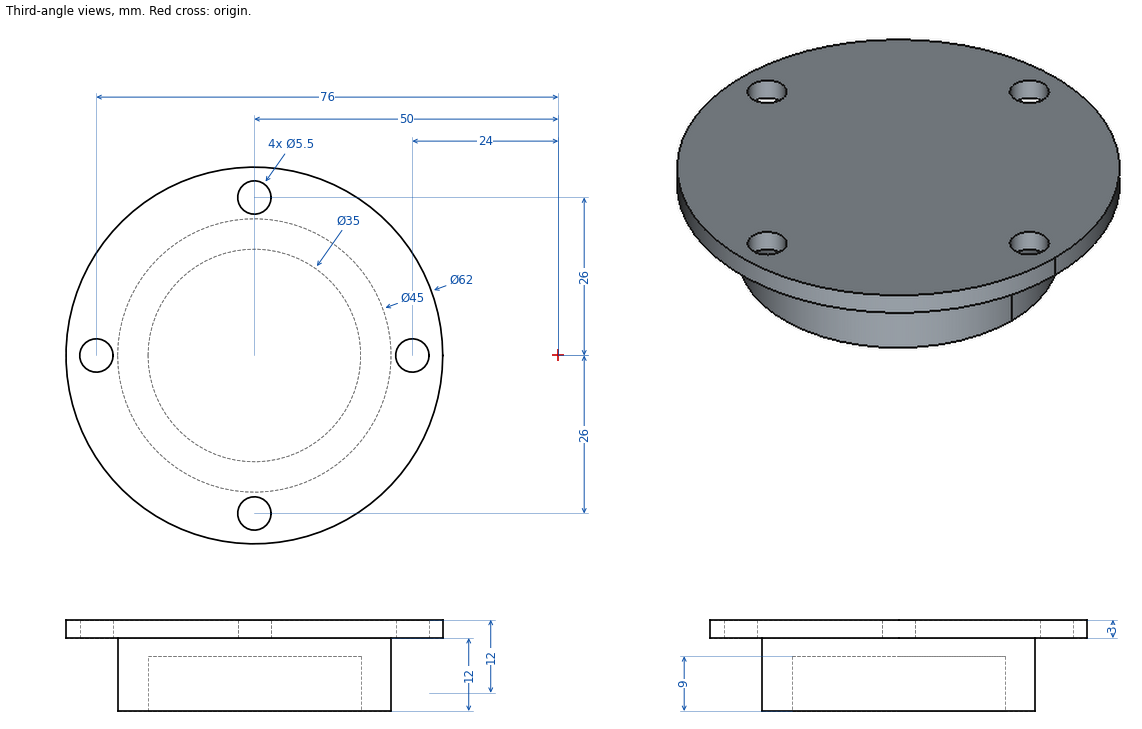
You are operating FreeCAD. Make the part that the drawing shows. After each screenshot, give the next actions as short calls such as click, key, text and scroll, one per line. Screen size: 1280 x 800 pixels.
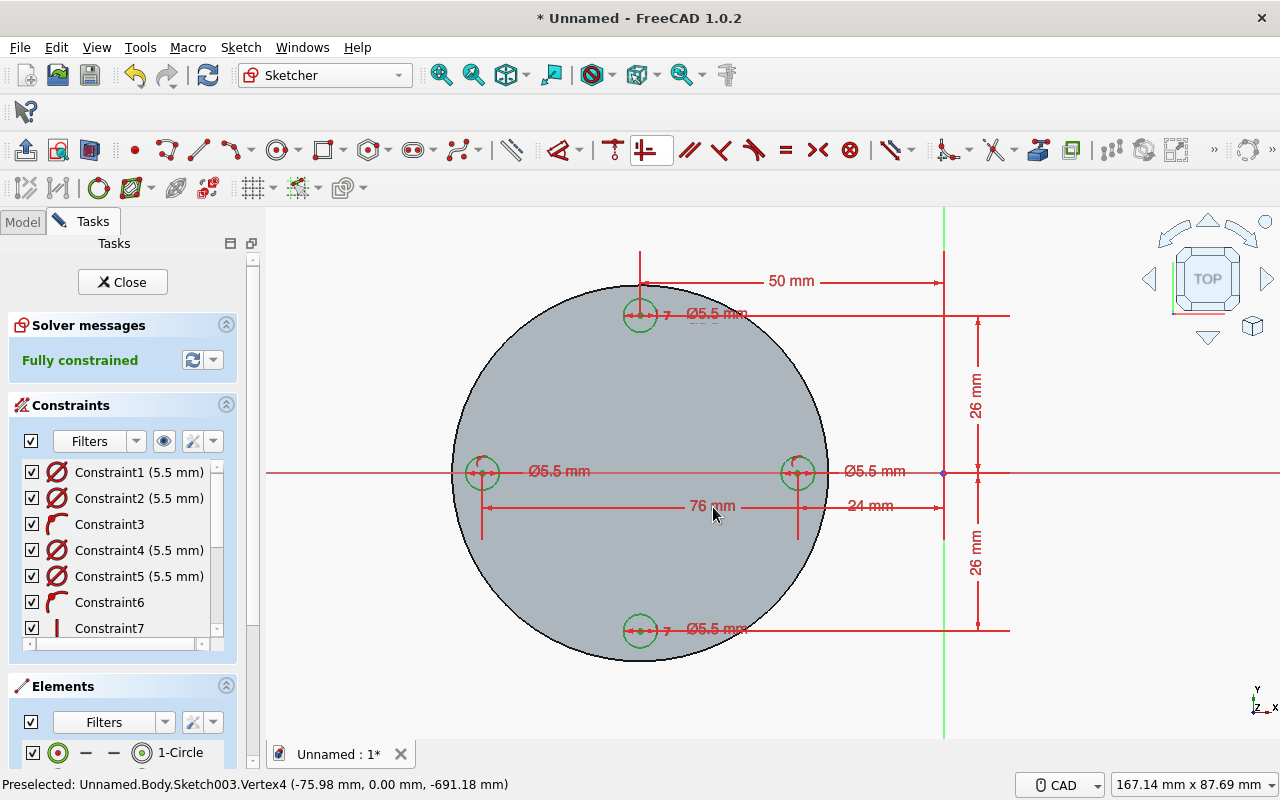
click(123, 282)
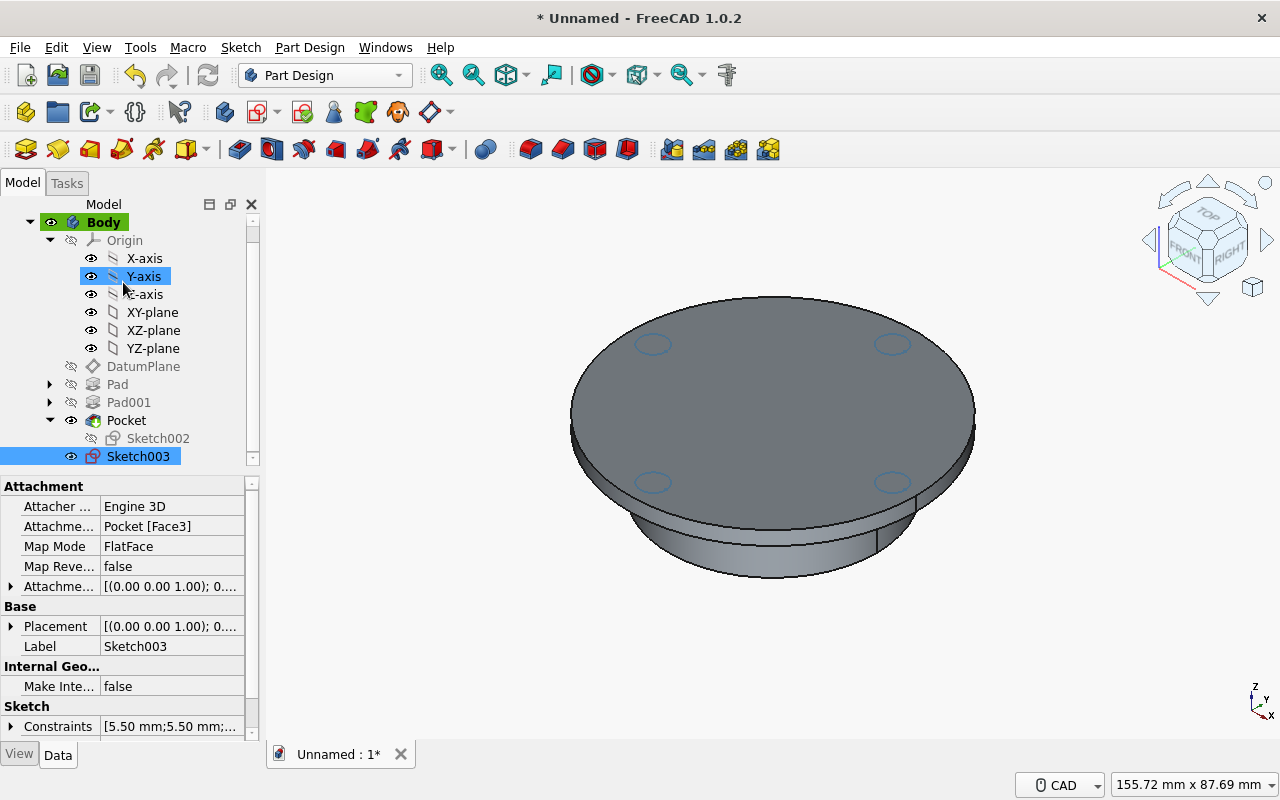
click(240, 150)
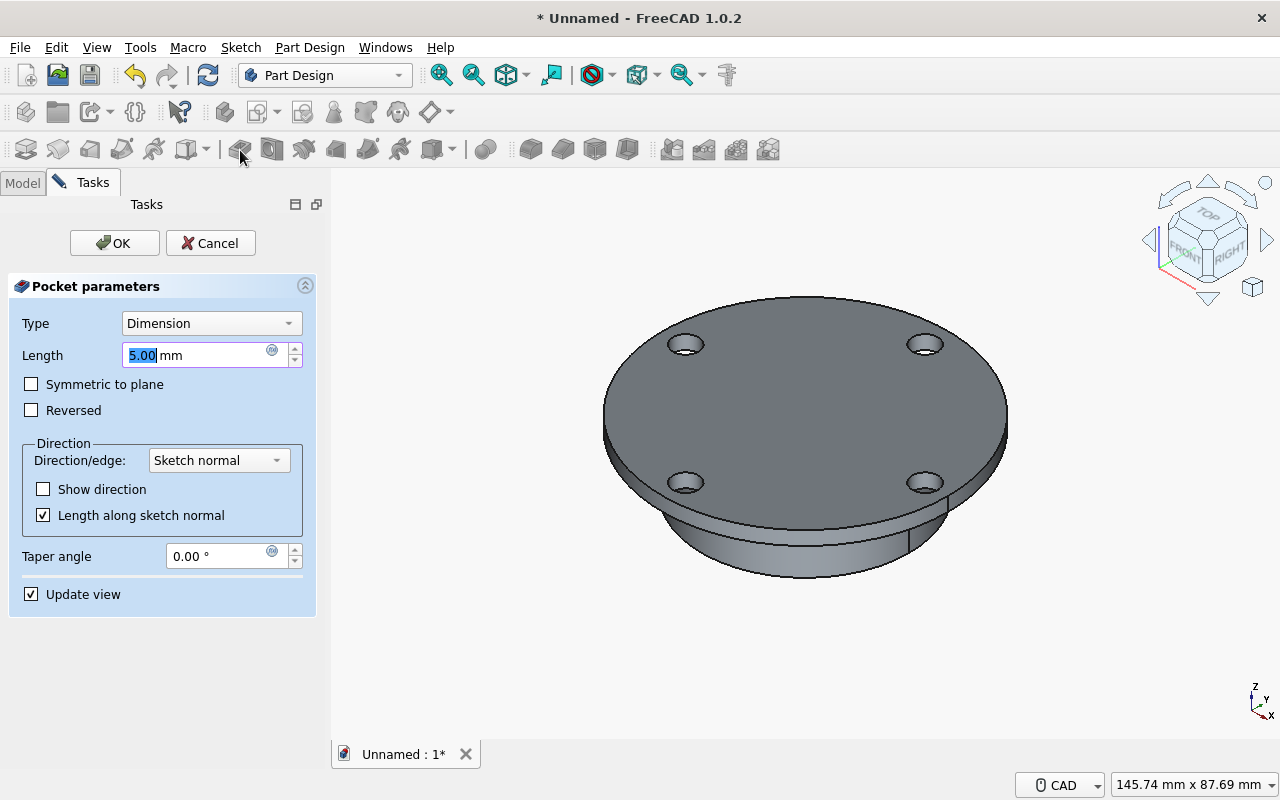
text(12)
key(Tab)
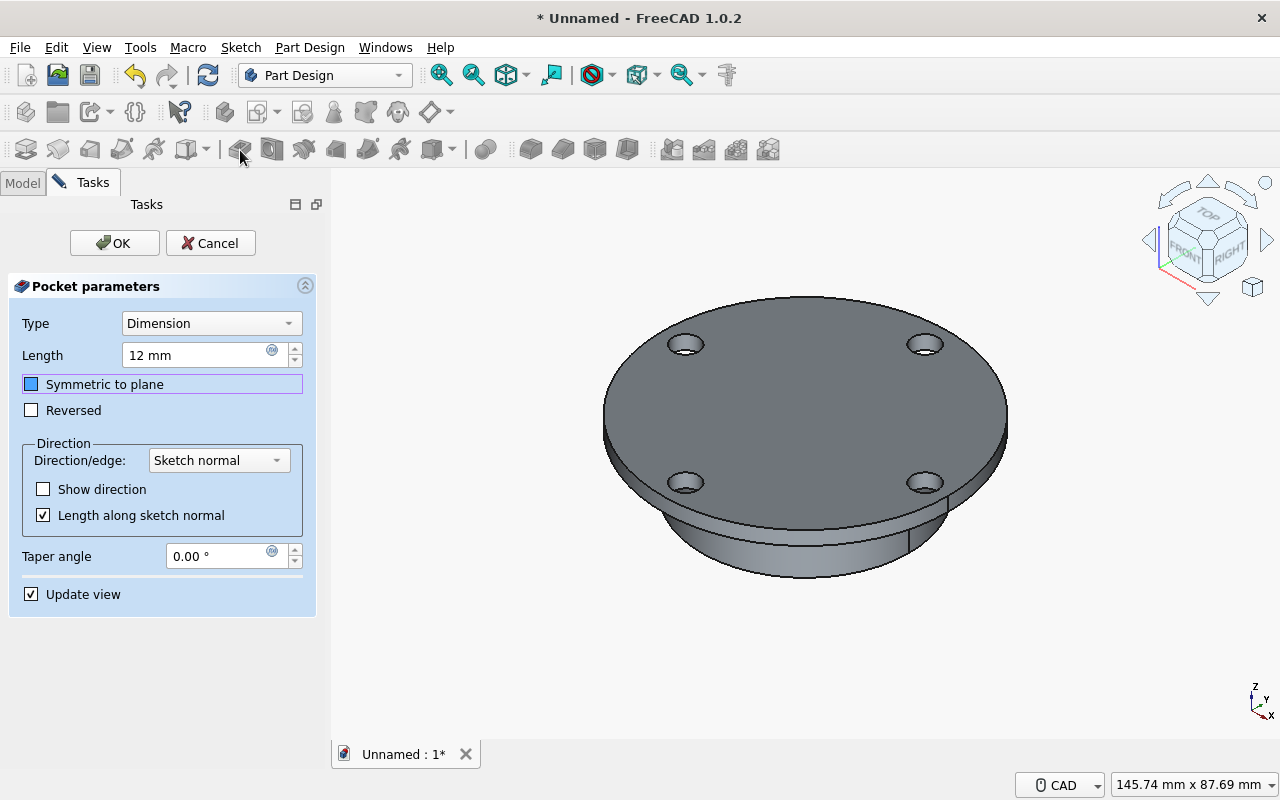
click(115, 243)